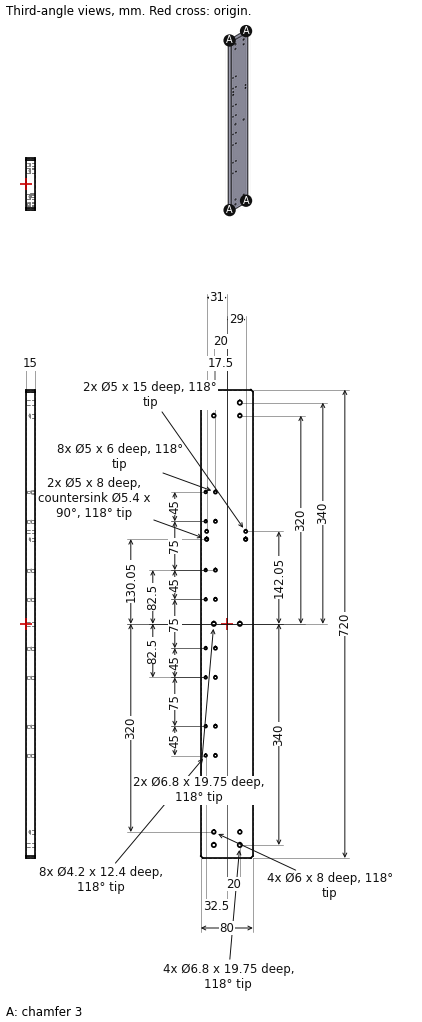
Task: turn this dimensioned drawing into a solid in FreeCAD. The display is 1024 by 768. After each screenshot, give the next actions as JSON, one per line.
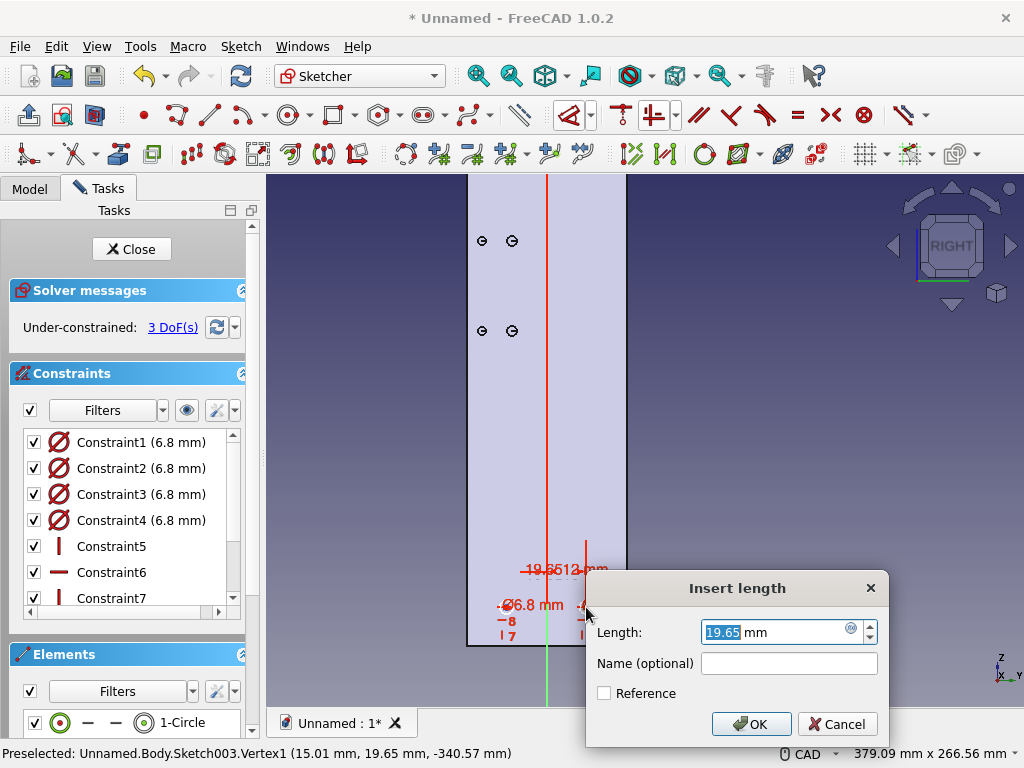
{"action": "type", "text": "20"}
{"action": "key", "text": "Return"}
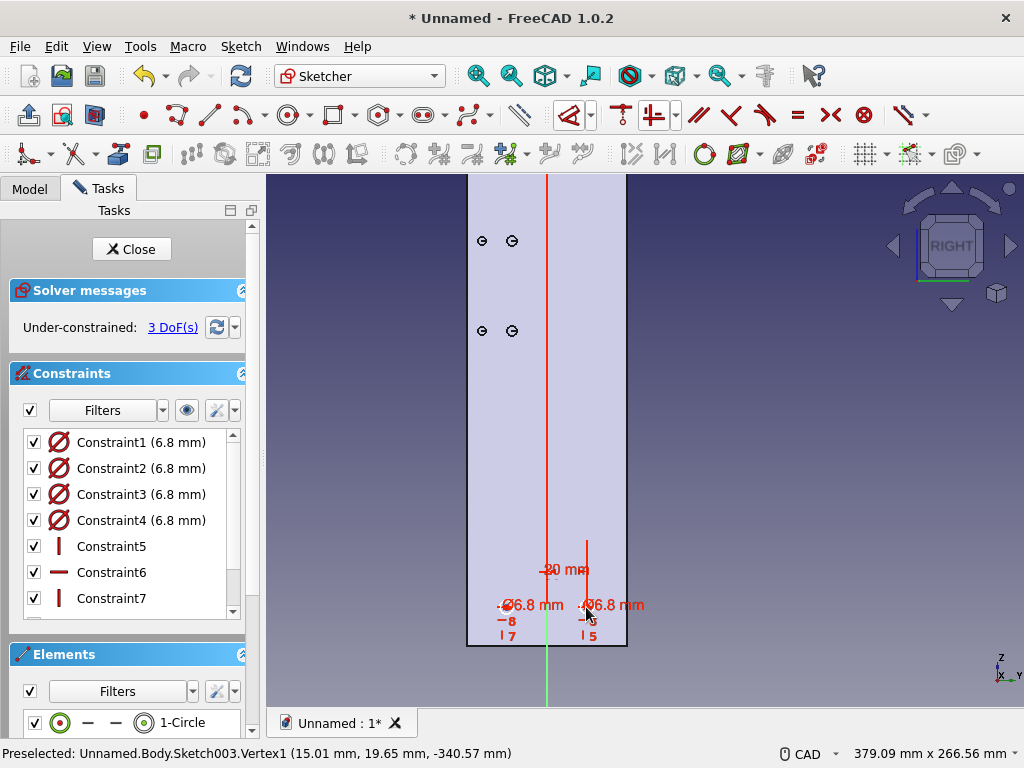
{"action": "scroll", "coordinate": [586, 609], "scroll_direction": "down", "scroll_amount": 7}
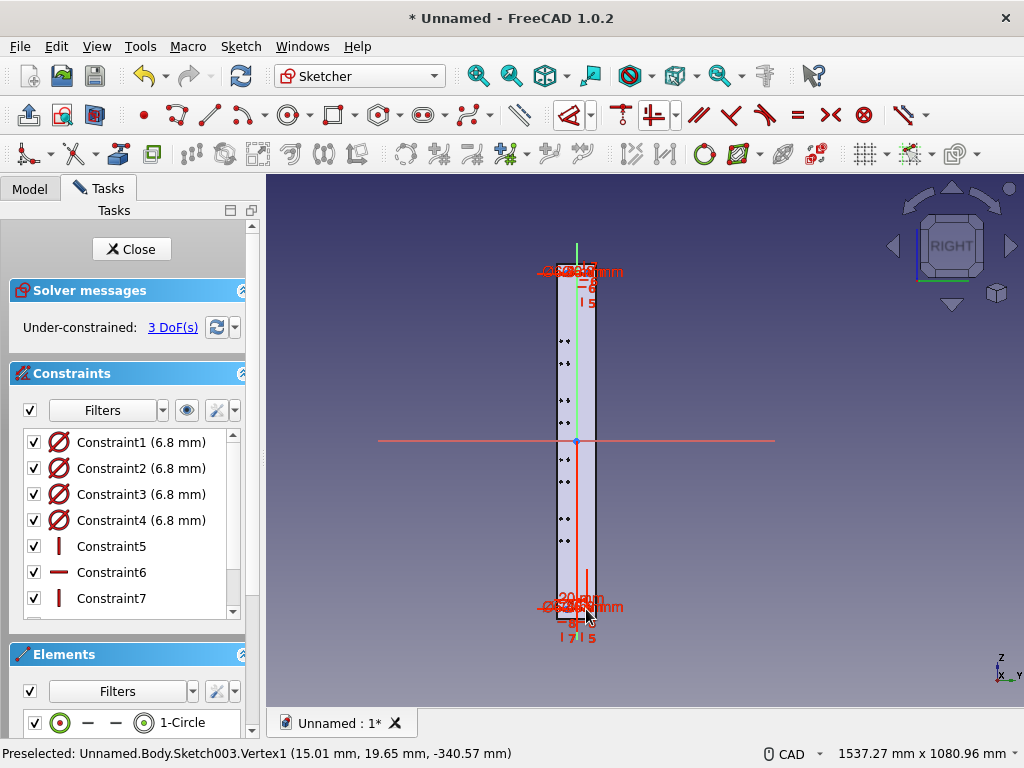
{"action": "scroll", "coordinate": [567, 274], "scroll_direction": "up", "scroll_amount": 7}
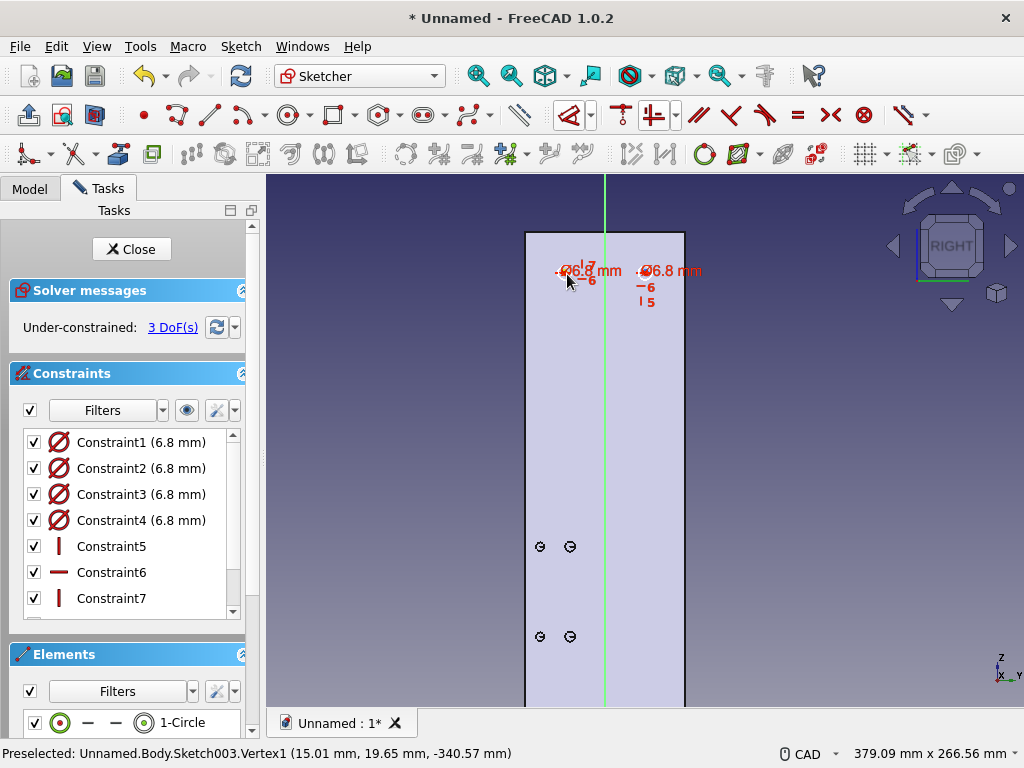
{"action": "left_click", "coordinate": [565, 273]}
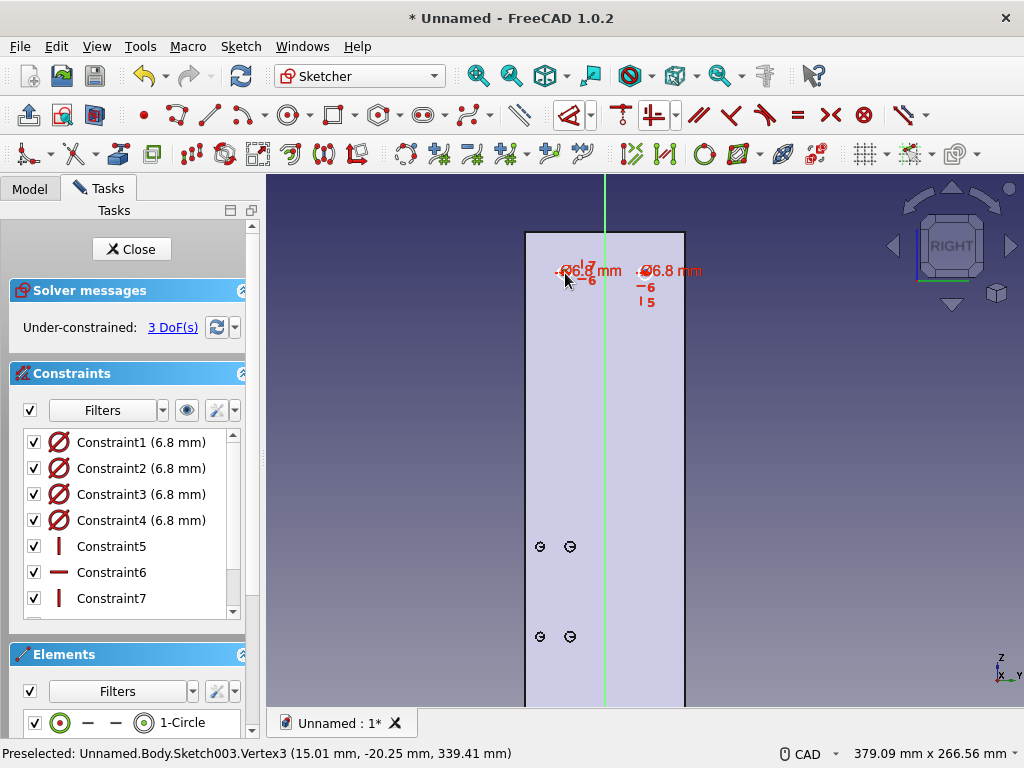
{"action": "key", "text": "l"}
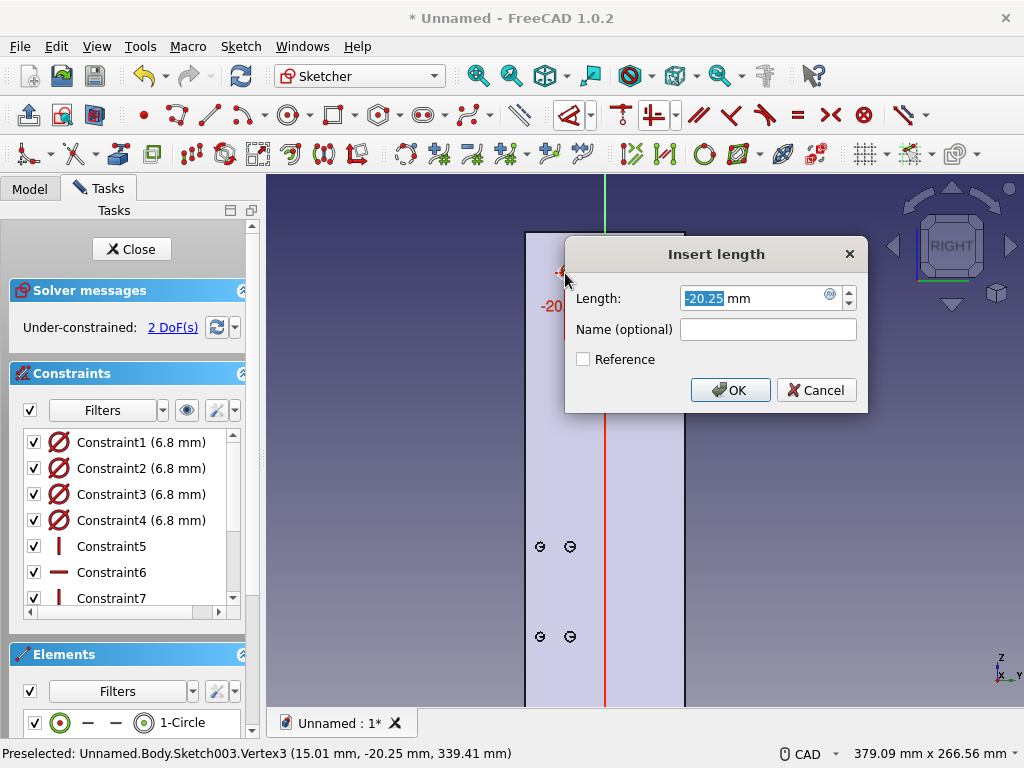
{"action": "type", "text": "-20"}
{"action": "key", "text": "Return"}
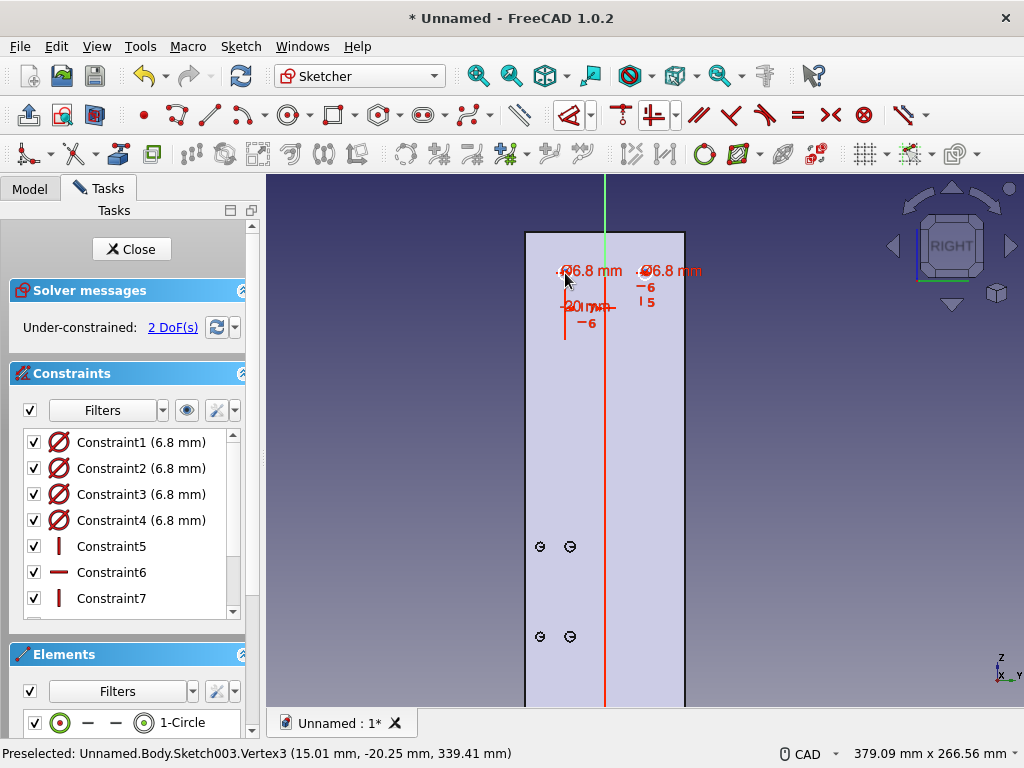
{"action": "scroll", "coordinate": [567, 273], "scroll_direction": "down", "scroll_amount": 7}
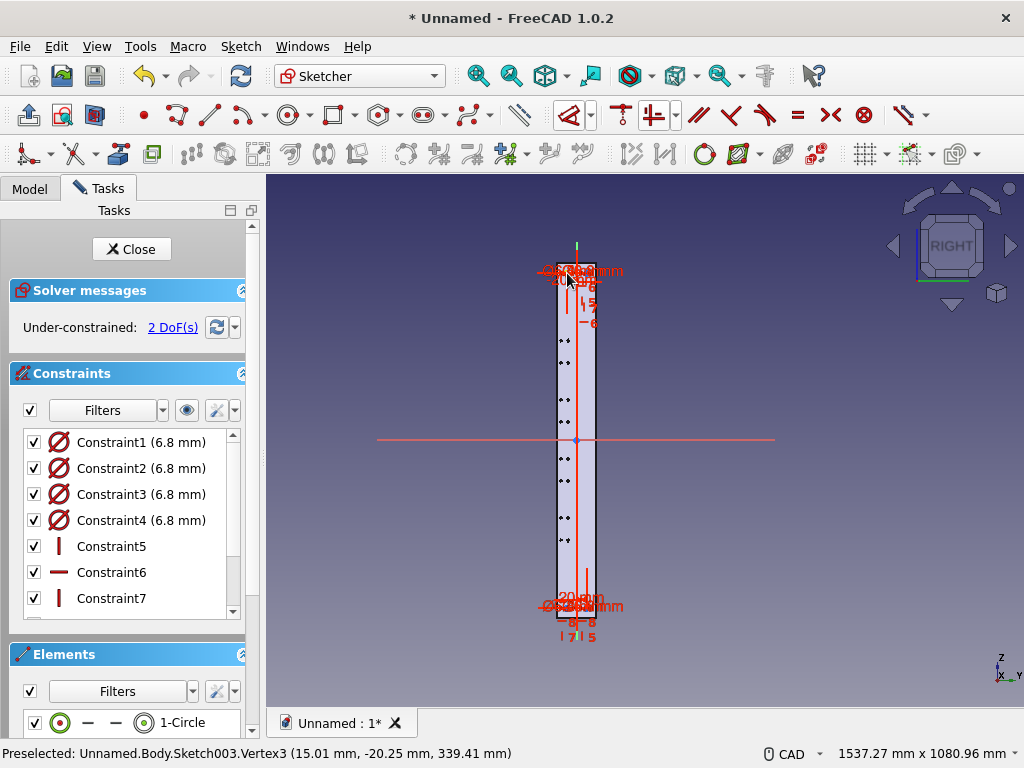
{"action": "left_click", "coordinate": [587, 608]}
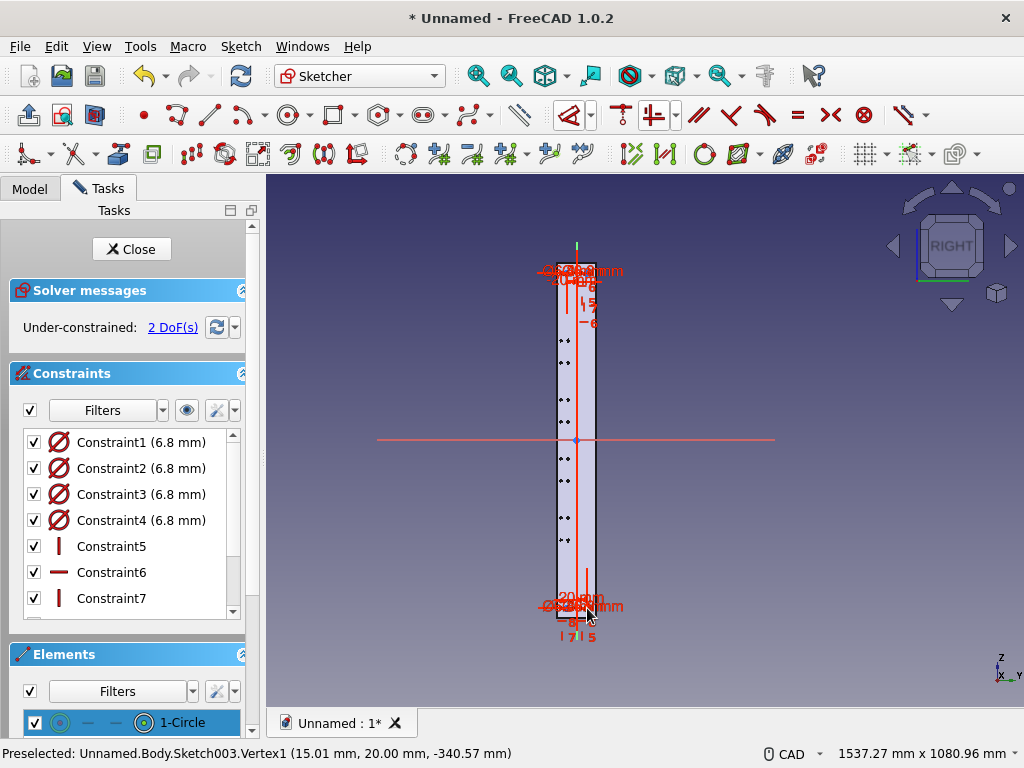
{"action": "key", "text": "i"}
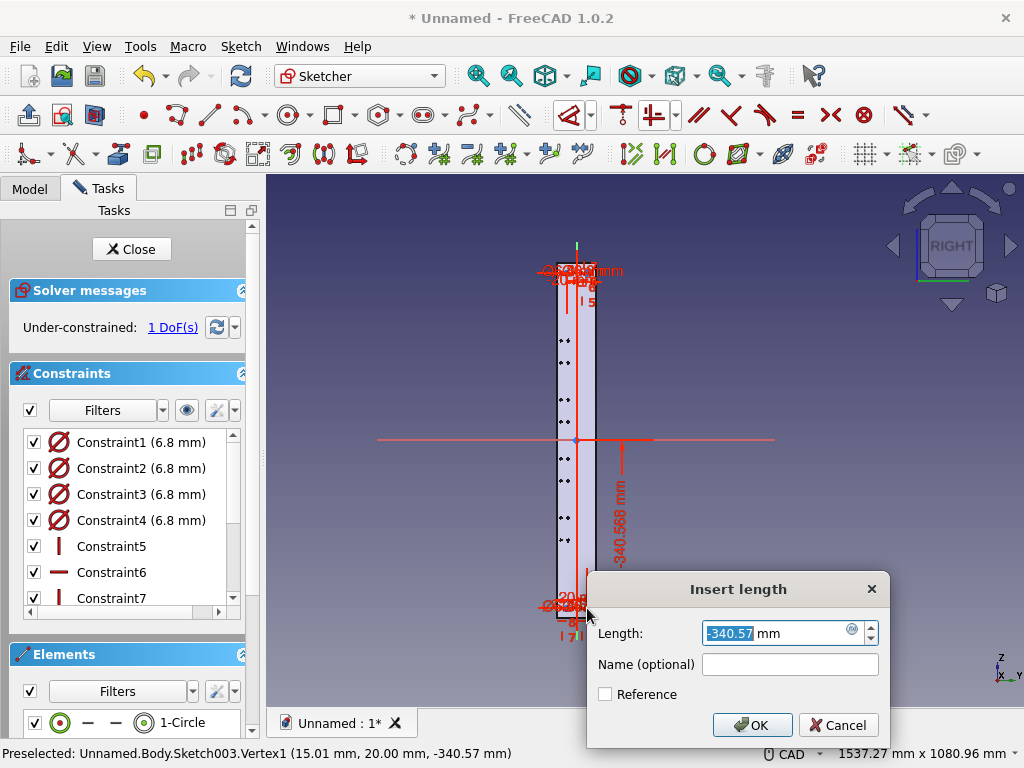
{"action": "type", "text": "-340"}
{"action": "key", "text": "Return"}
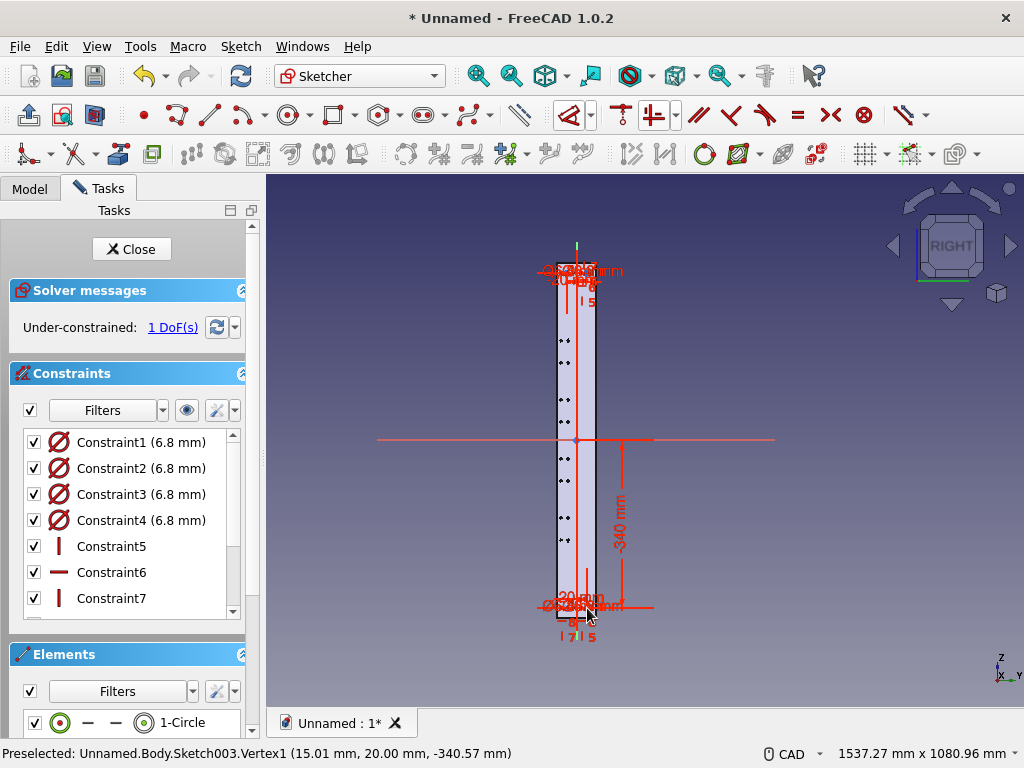
{"action": "left_click", "coordinate": [587, 273]}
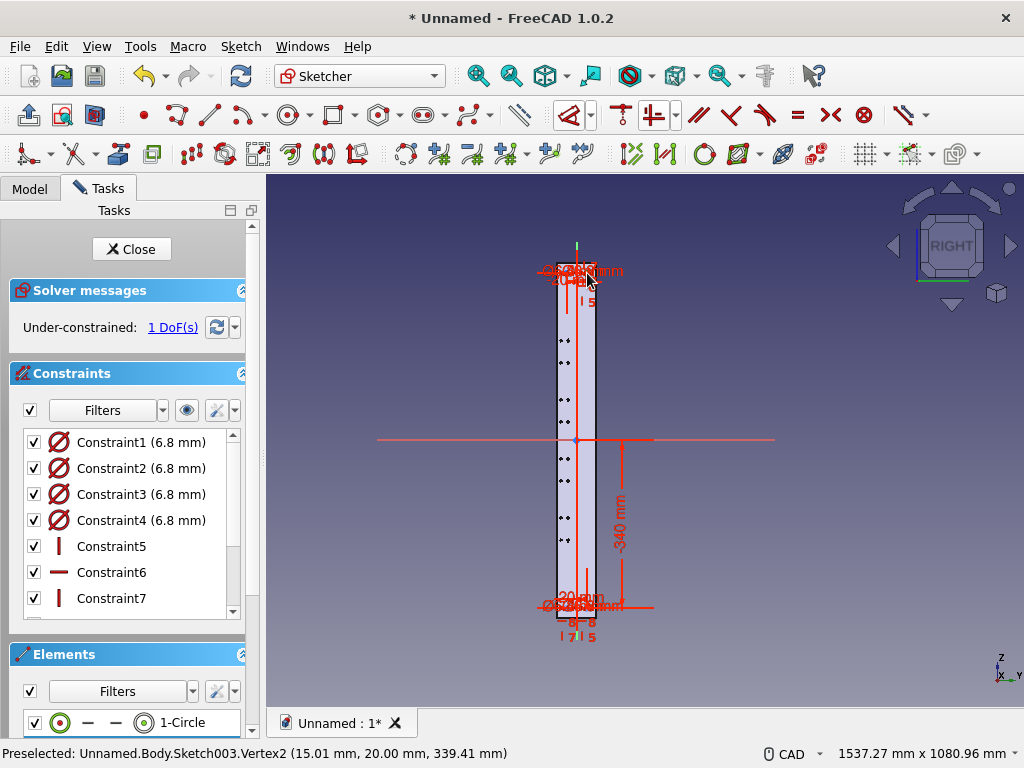
{"action": "key", "text": "i"}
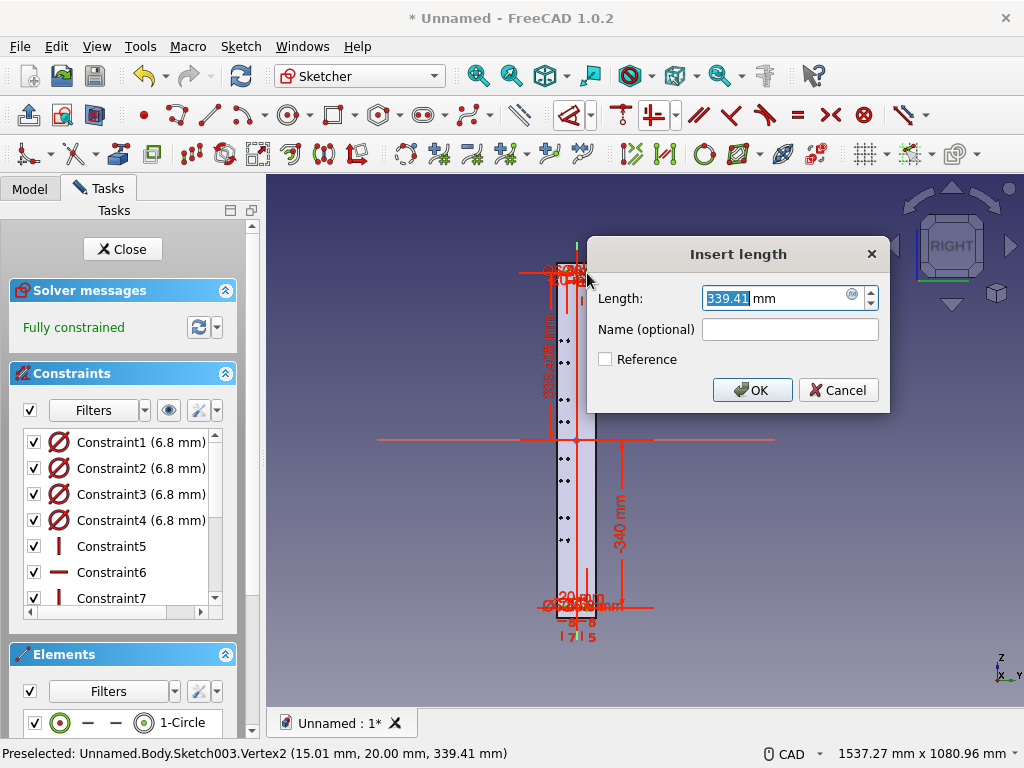
{"action": "type", "text": "340"}
{"action": "key", "text": "Return"}